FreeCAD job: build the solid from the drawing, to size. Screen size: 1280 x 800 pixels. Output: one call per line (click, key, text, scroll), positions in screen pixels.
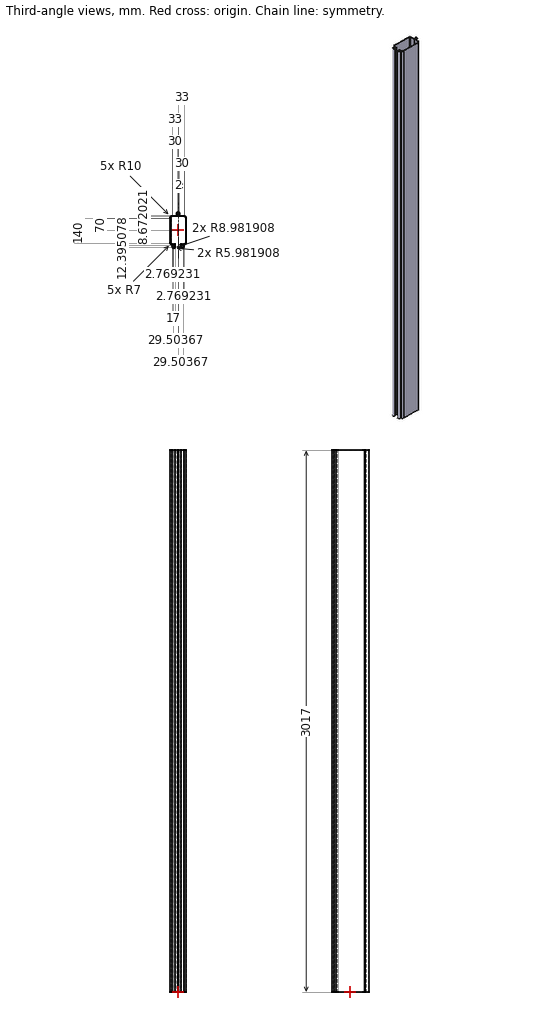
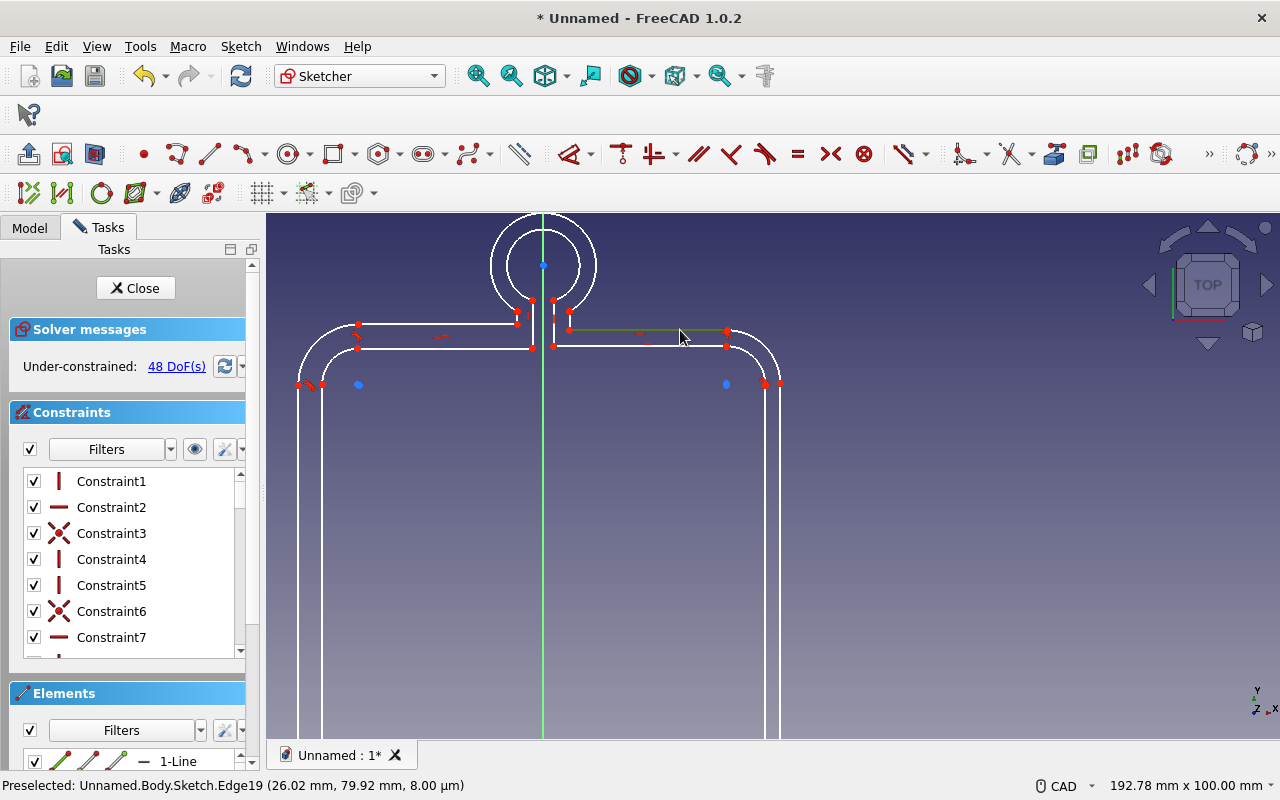
click(774, 360)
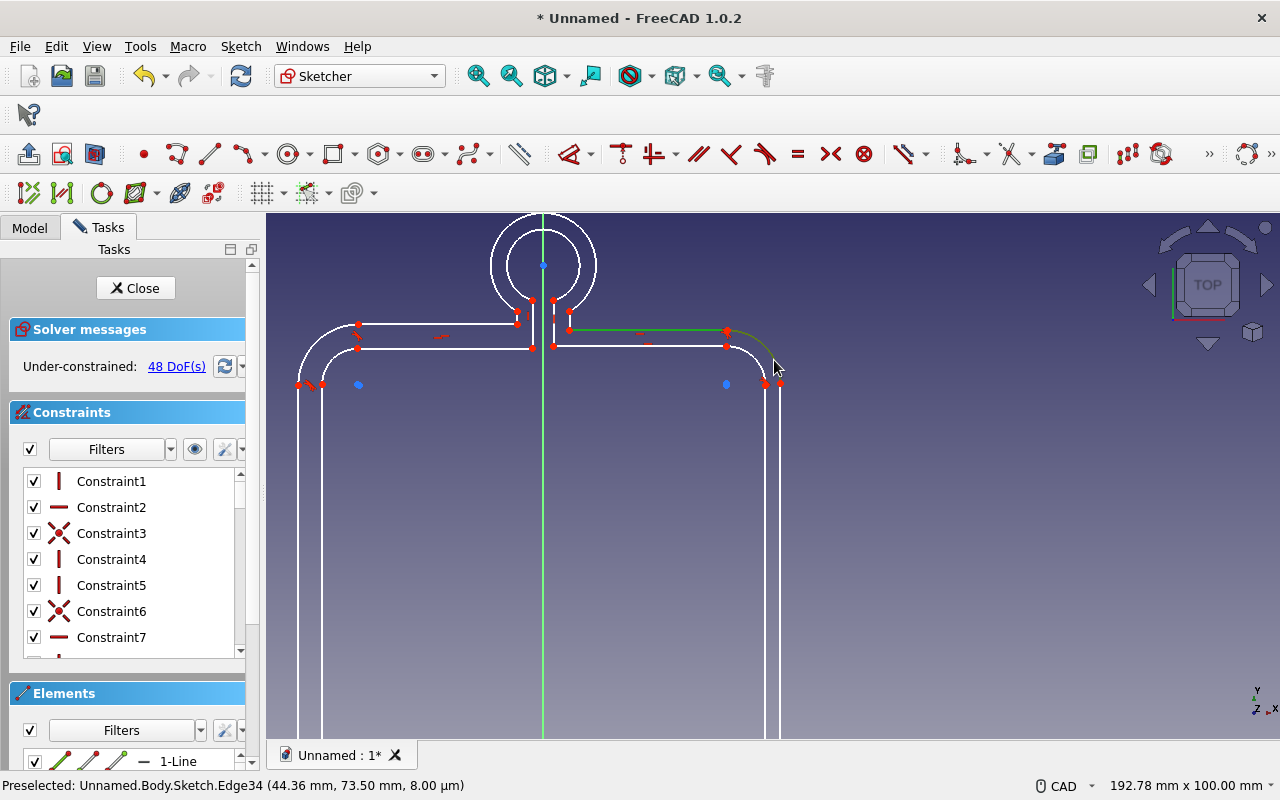
click(765, 154)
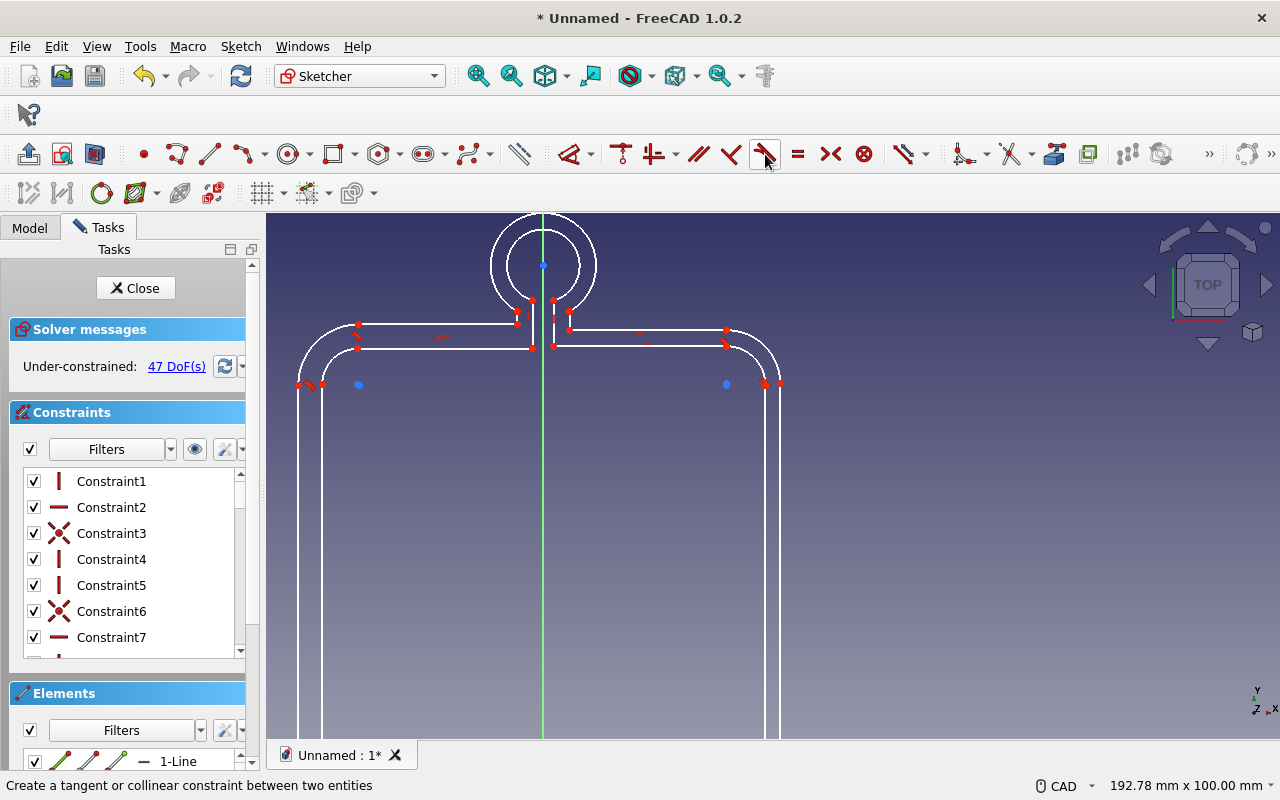
click(470, 324)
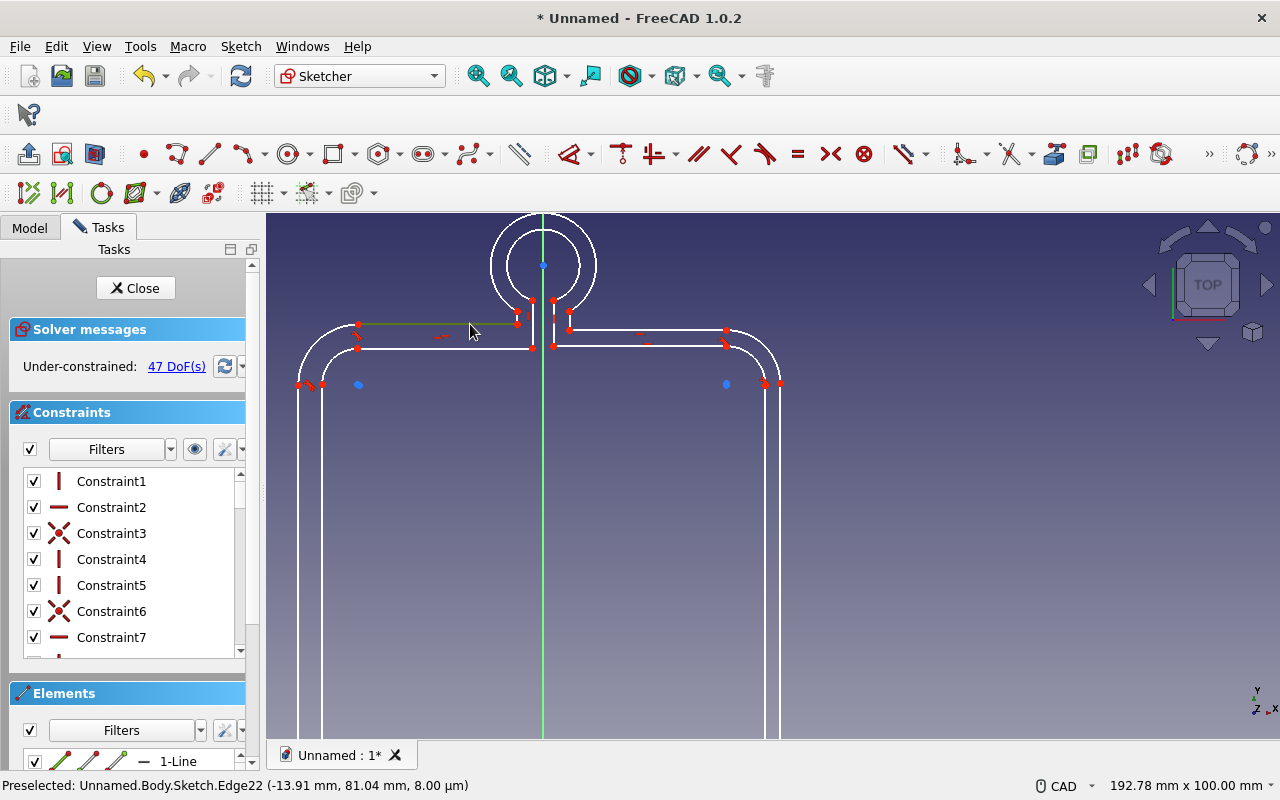
click(331, 331)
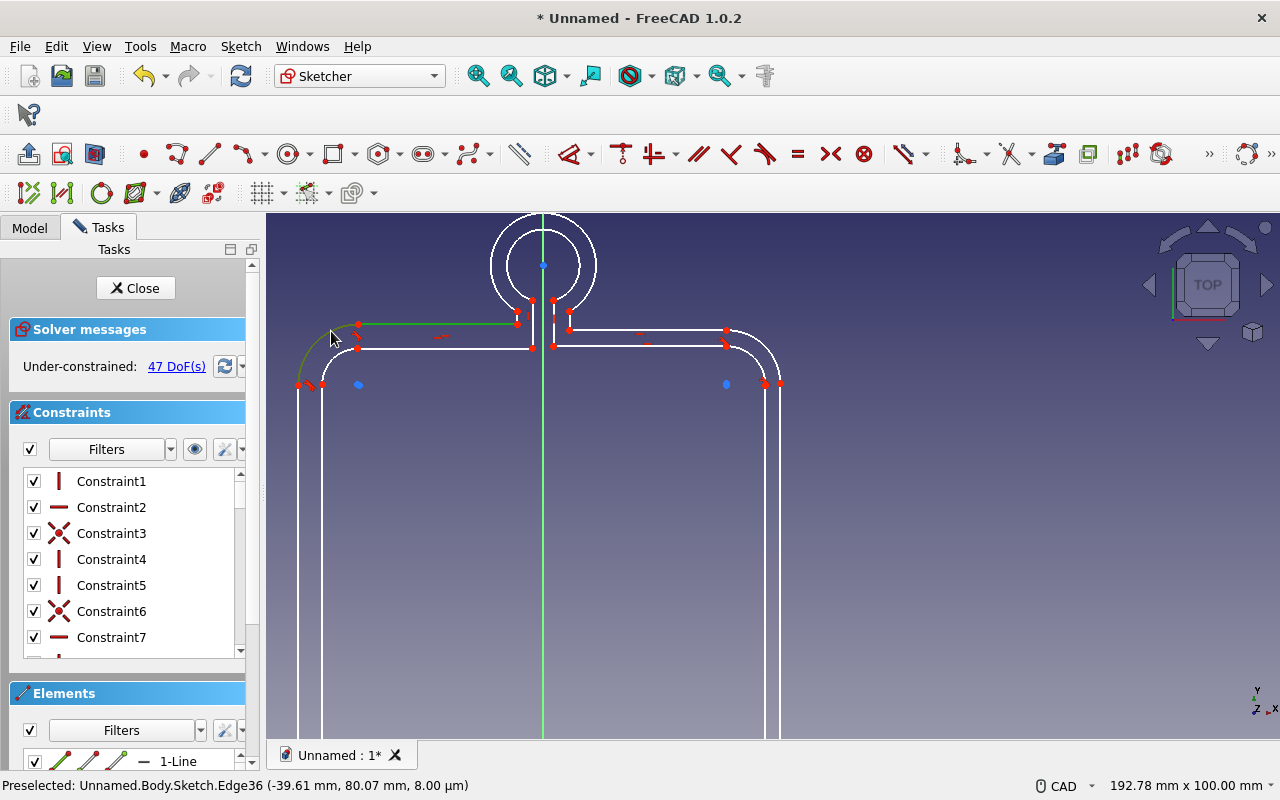
click(765, 154)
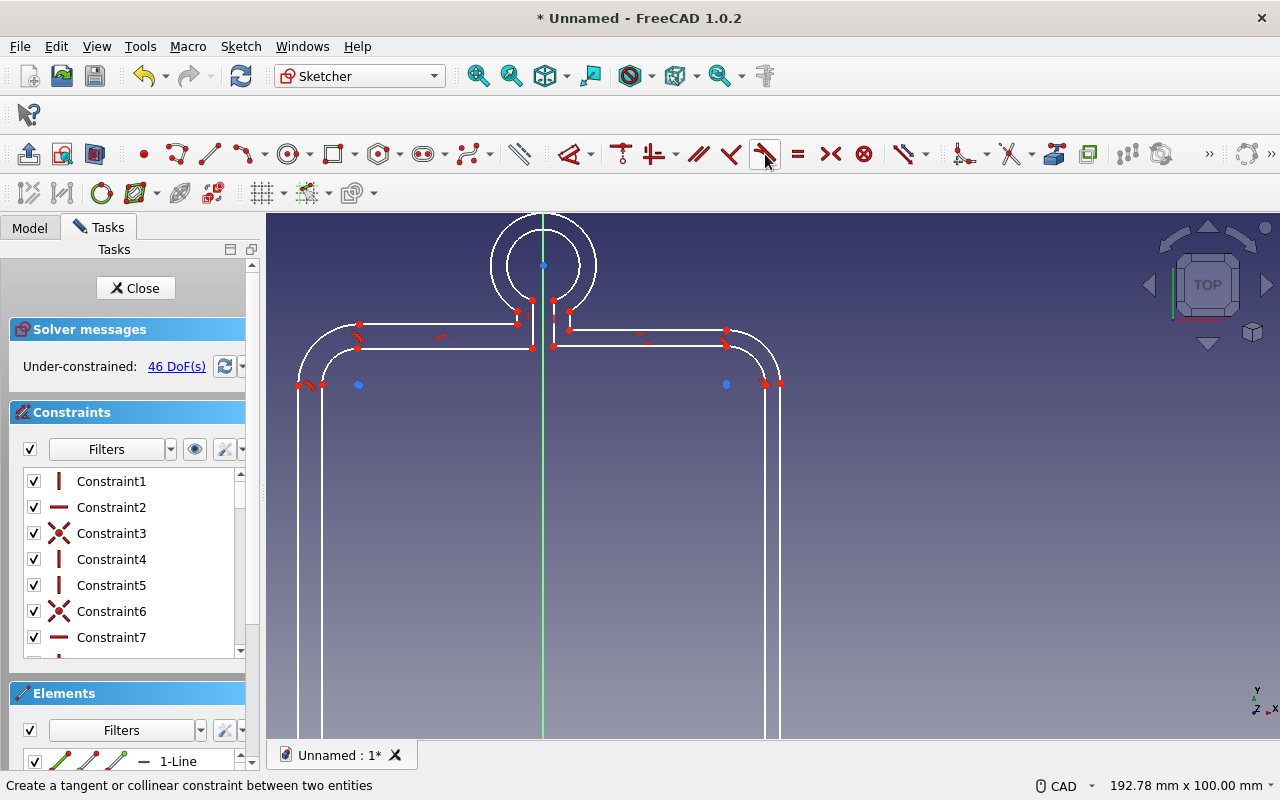
scroll(774, 359, down, 6)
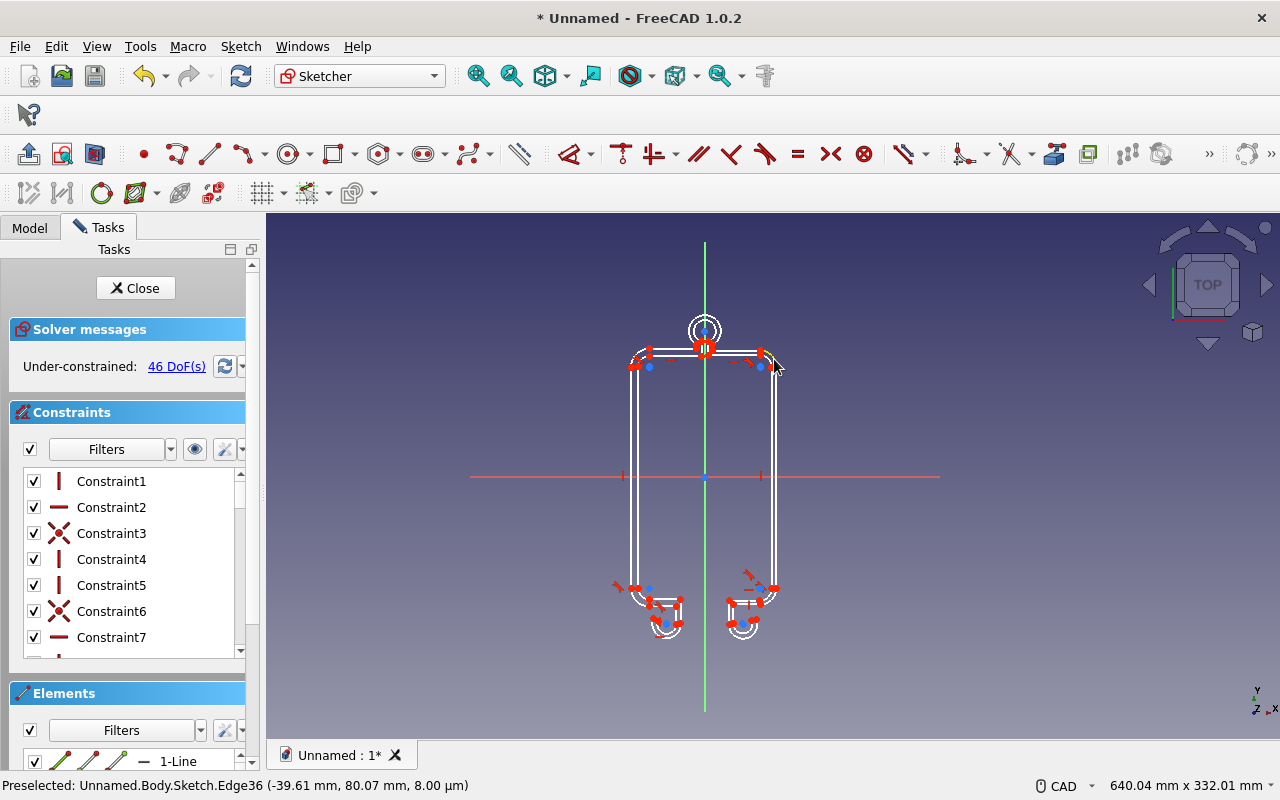
scroll(659, 630, up, 6)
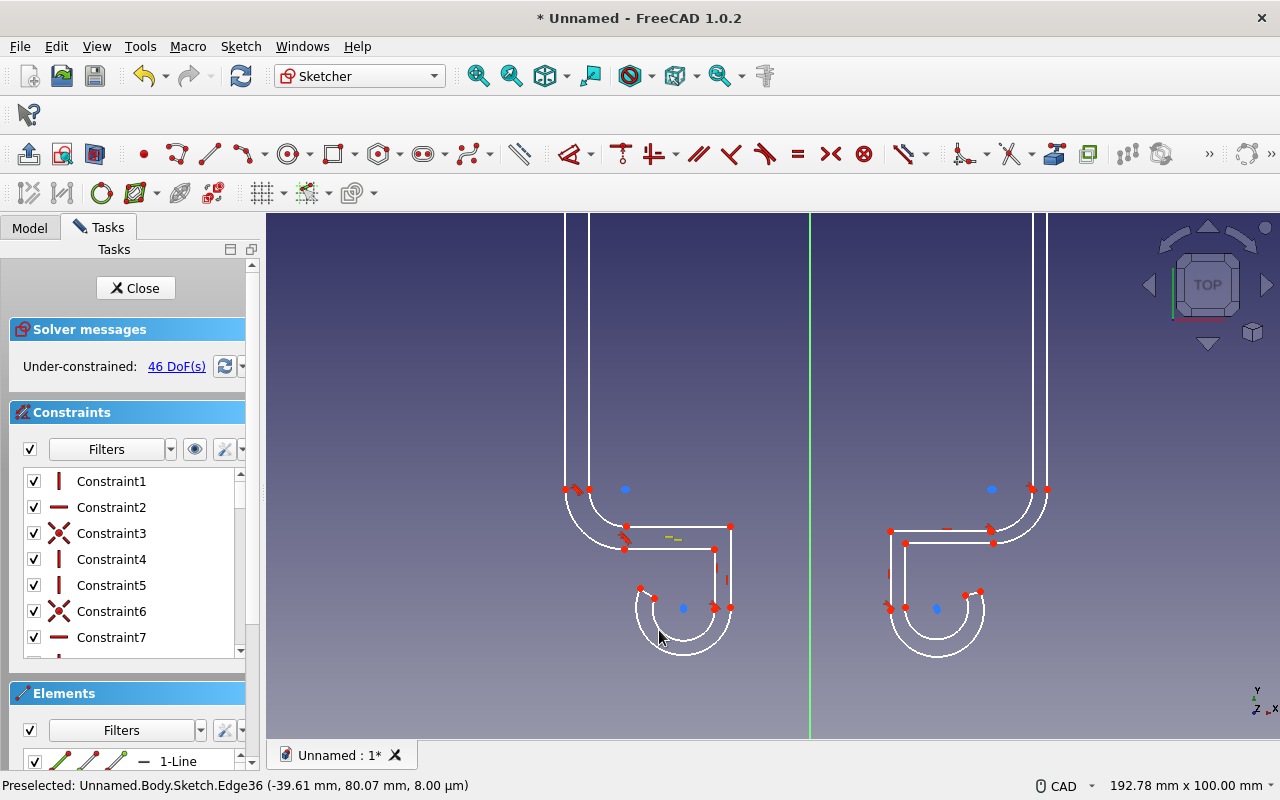
click(660, 629)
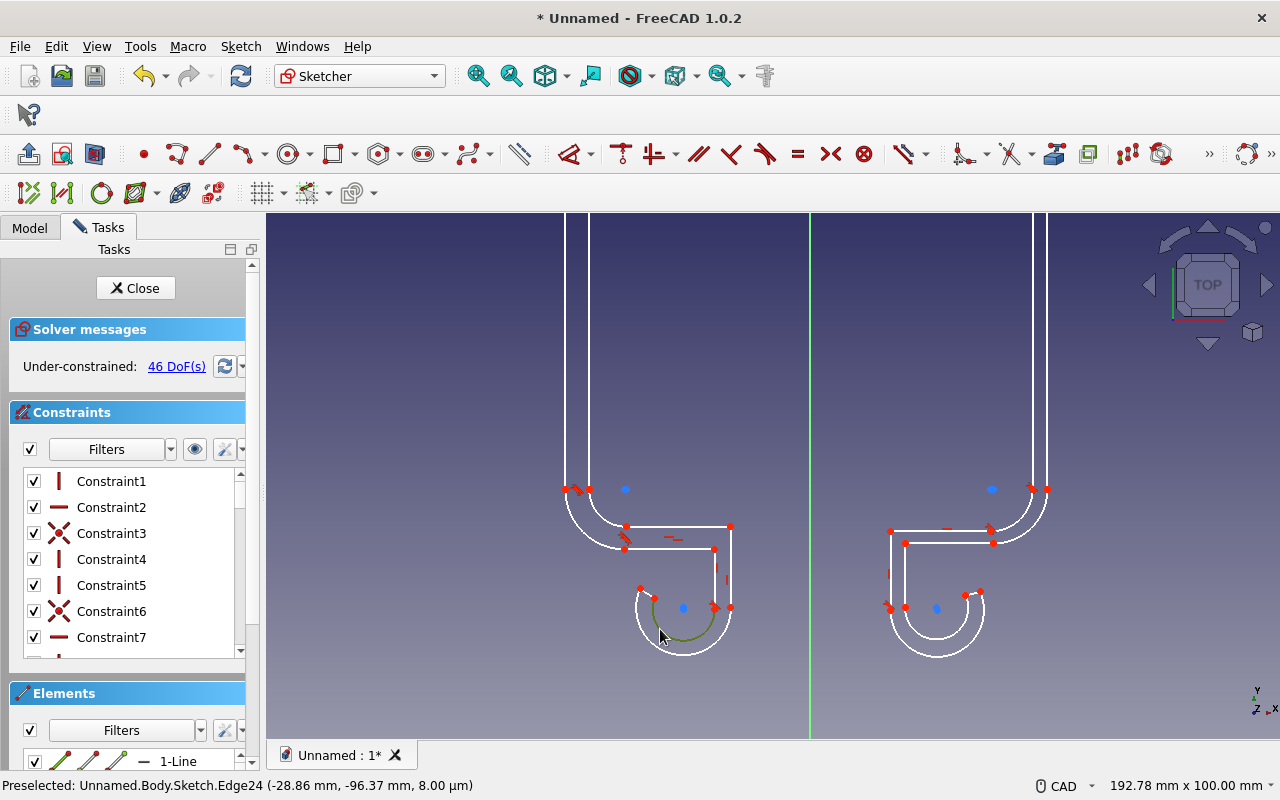
click(646, 637)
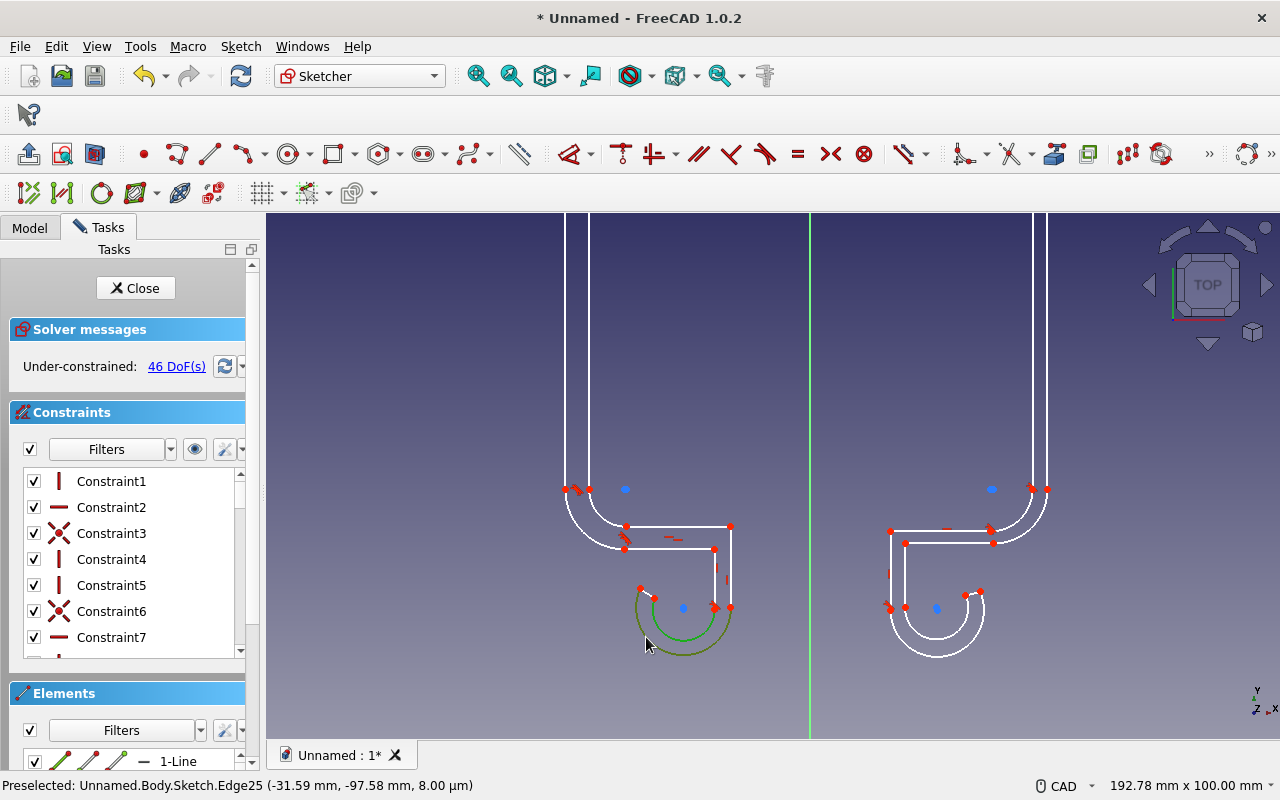
click(621, 154)